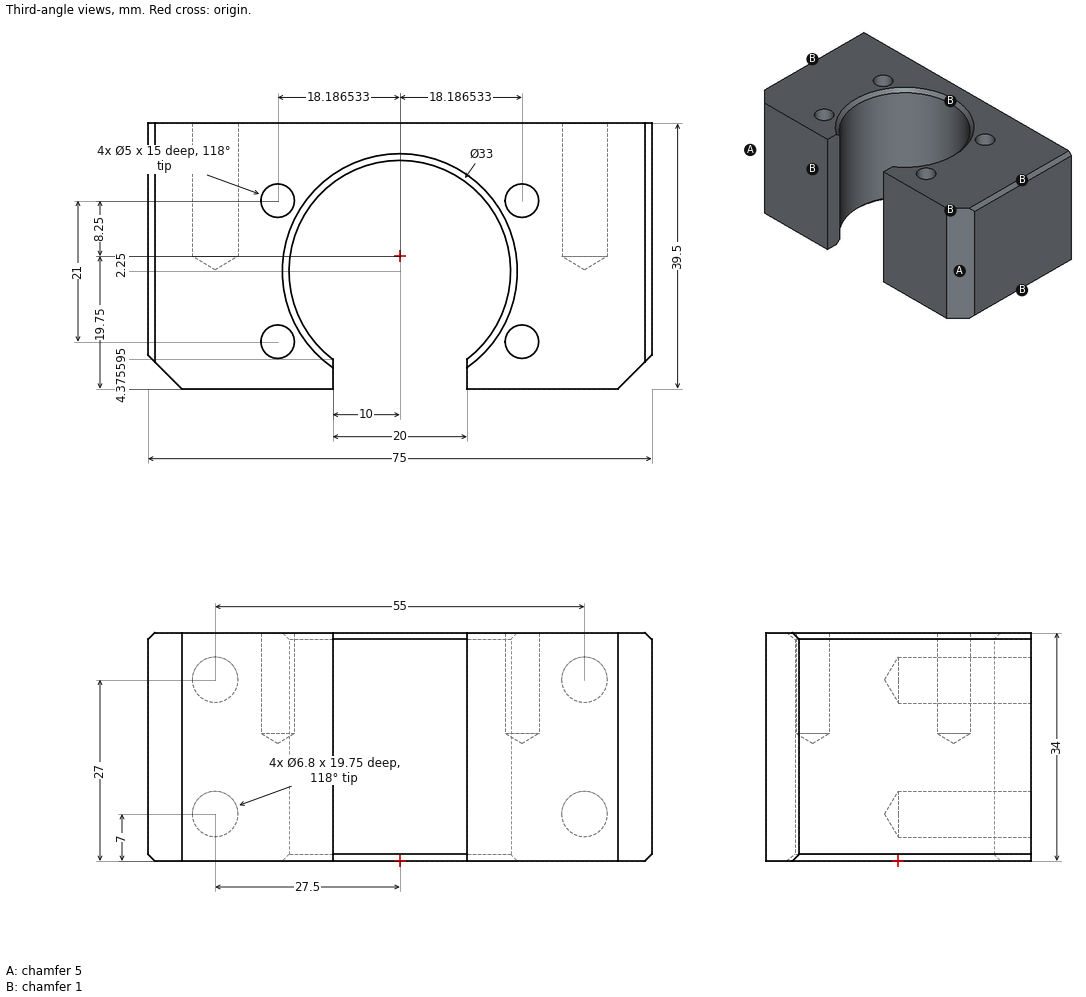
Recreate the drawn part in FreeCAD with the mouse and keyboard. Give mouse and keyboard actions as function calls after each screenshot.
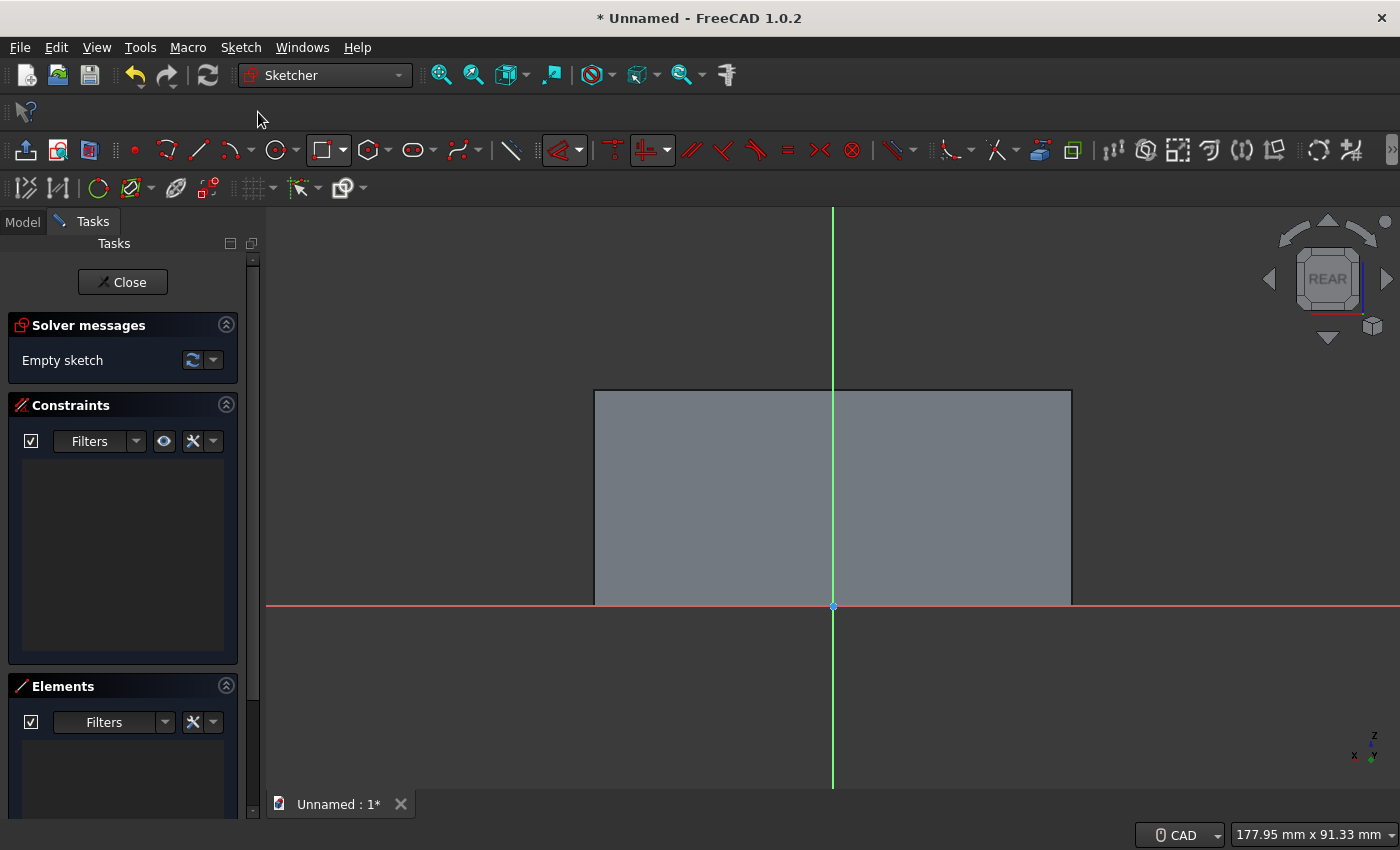
scroll(916, 523, up, 3)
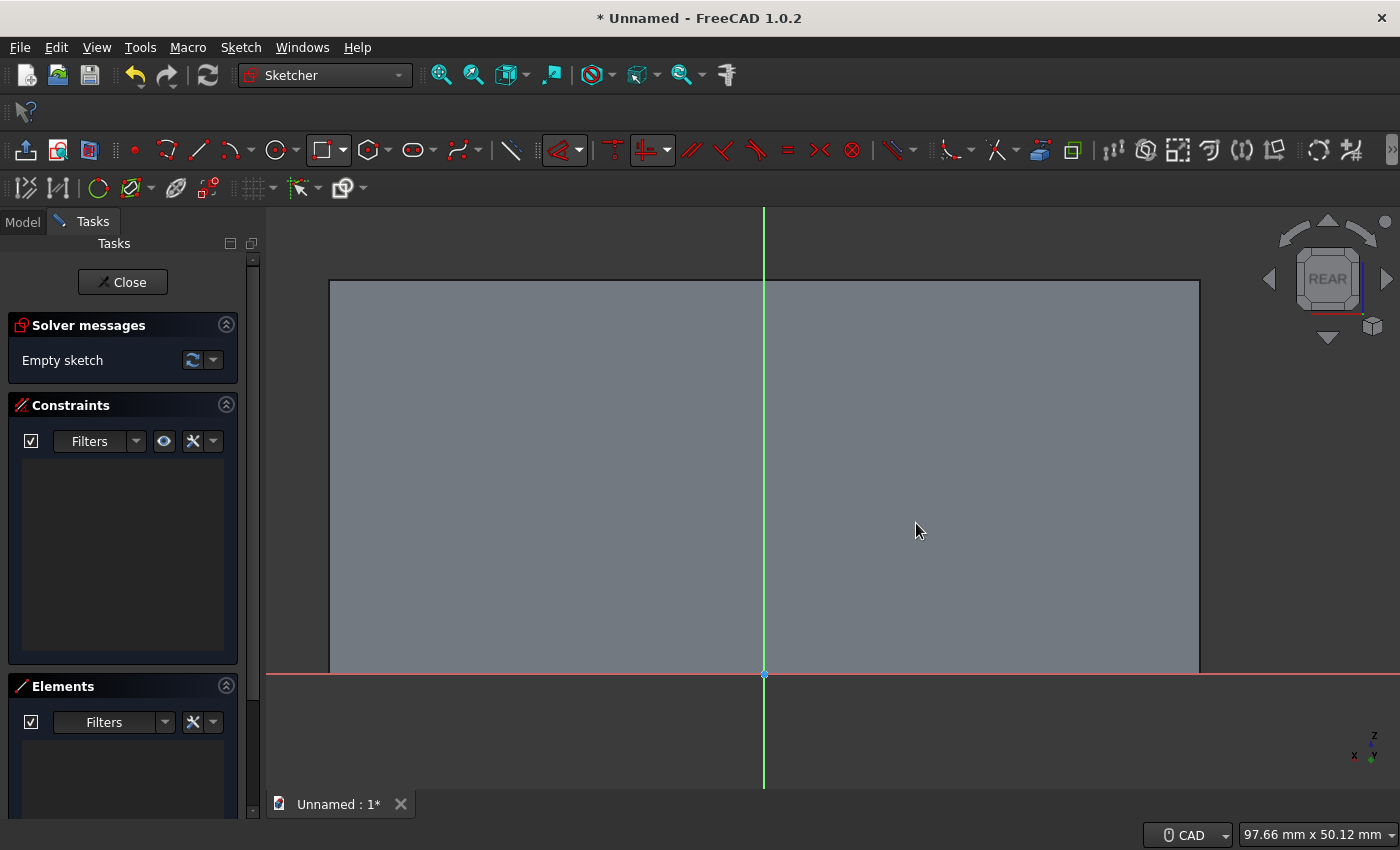
key(g)
key(c)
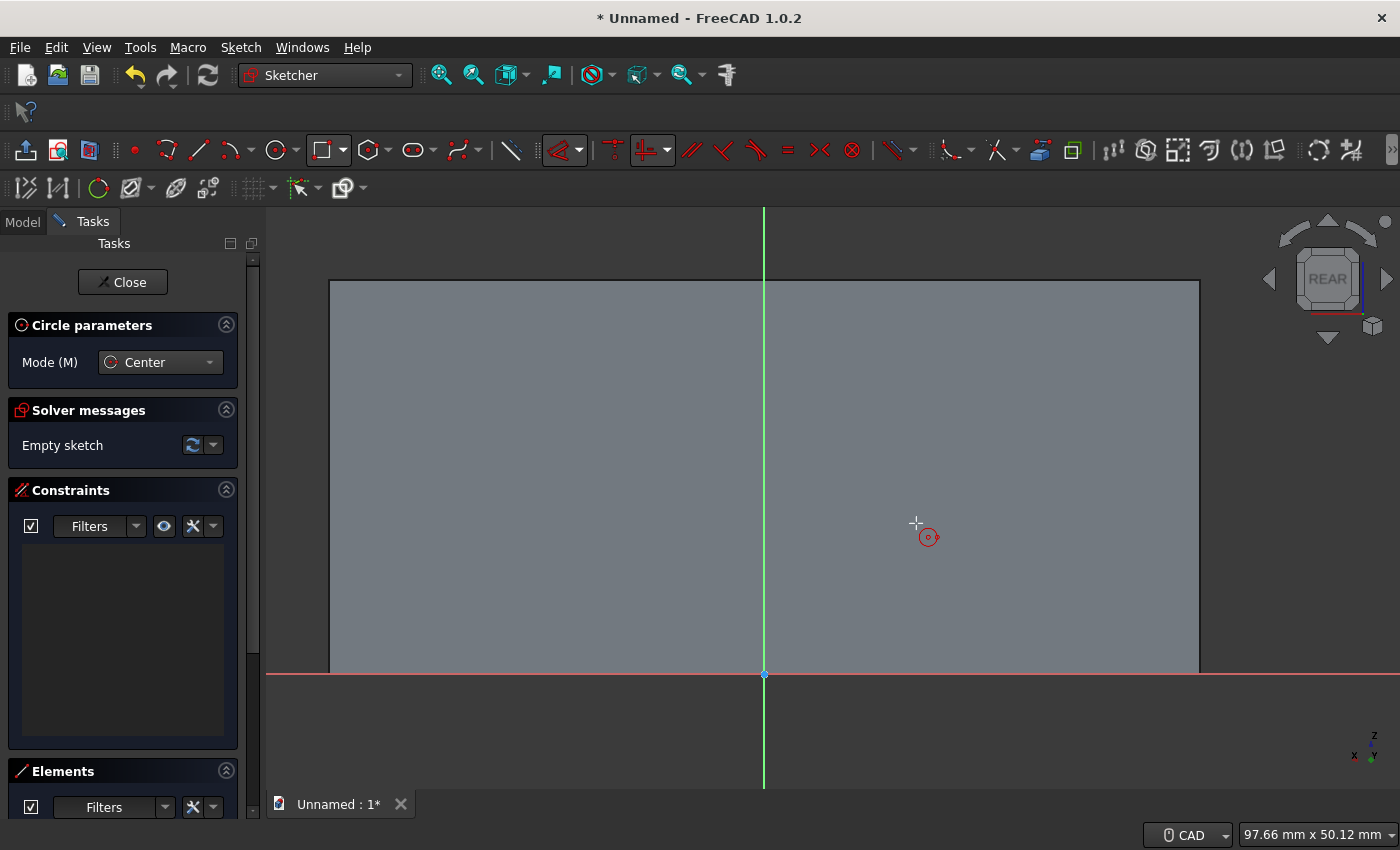
click(1084, 593)
click(1112, 565)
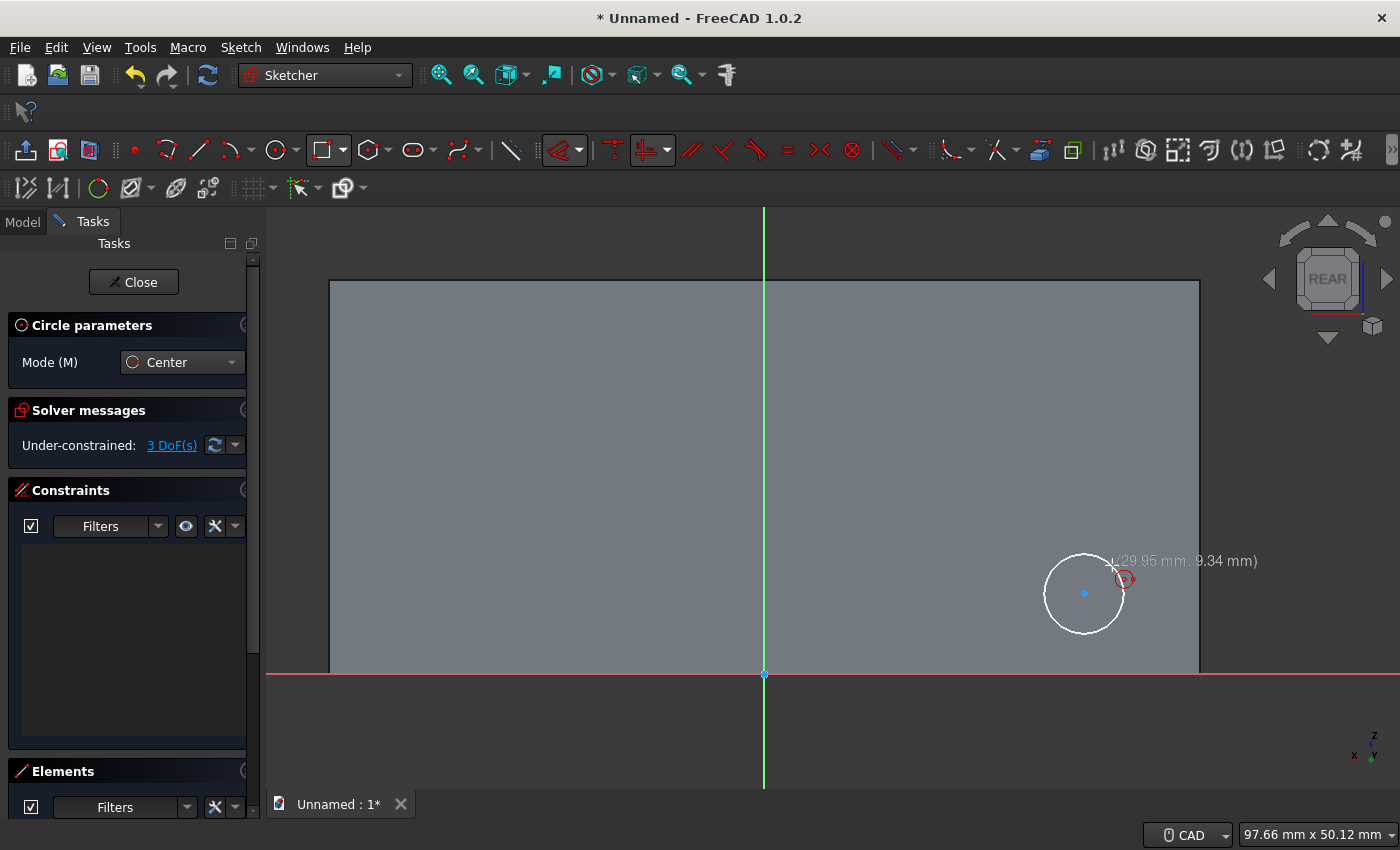
click(1084, 361)
click(1112, 333)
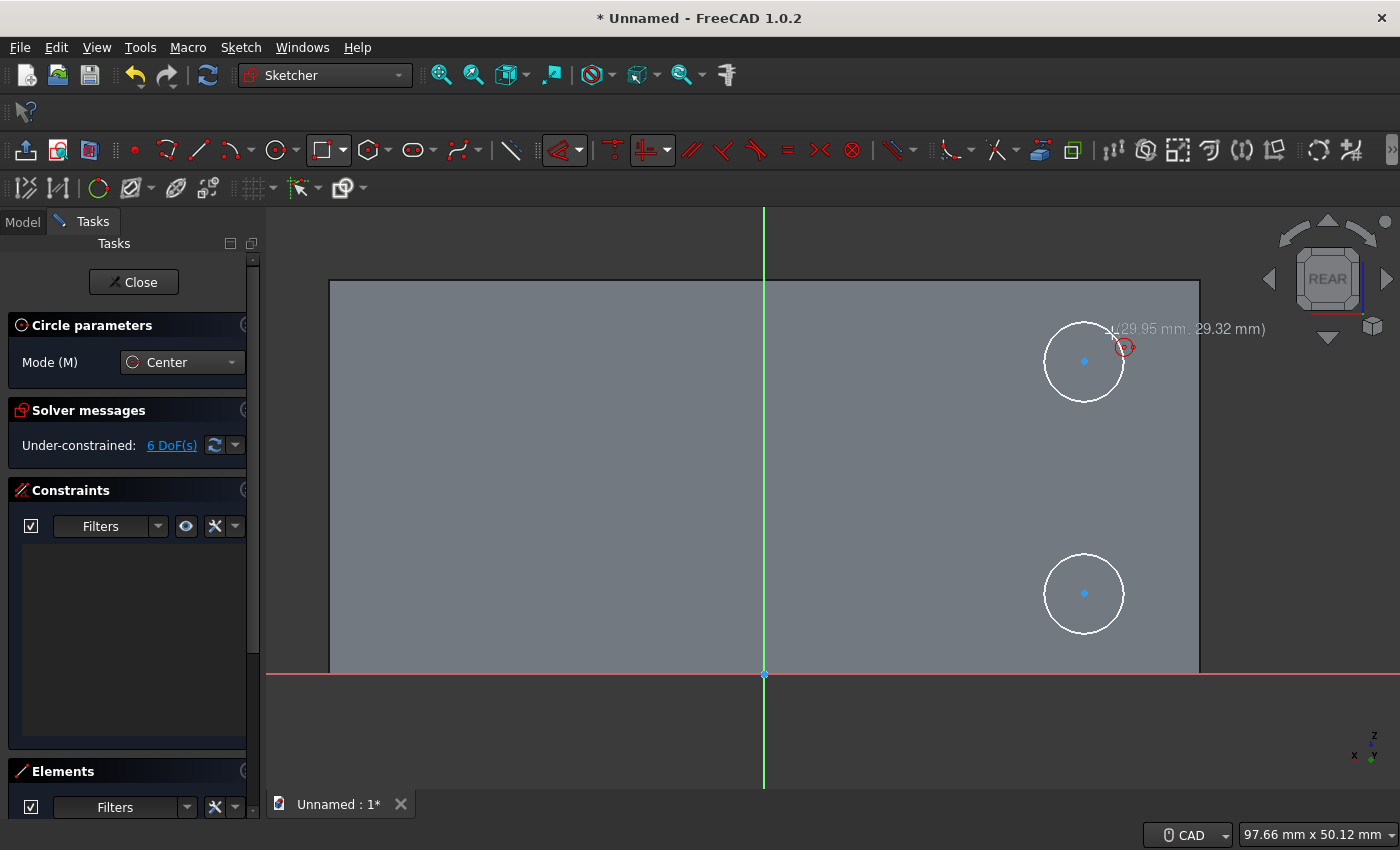
click(445, 361)
click(473, 333)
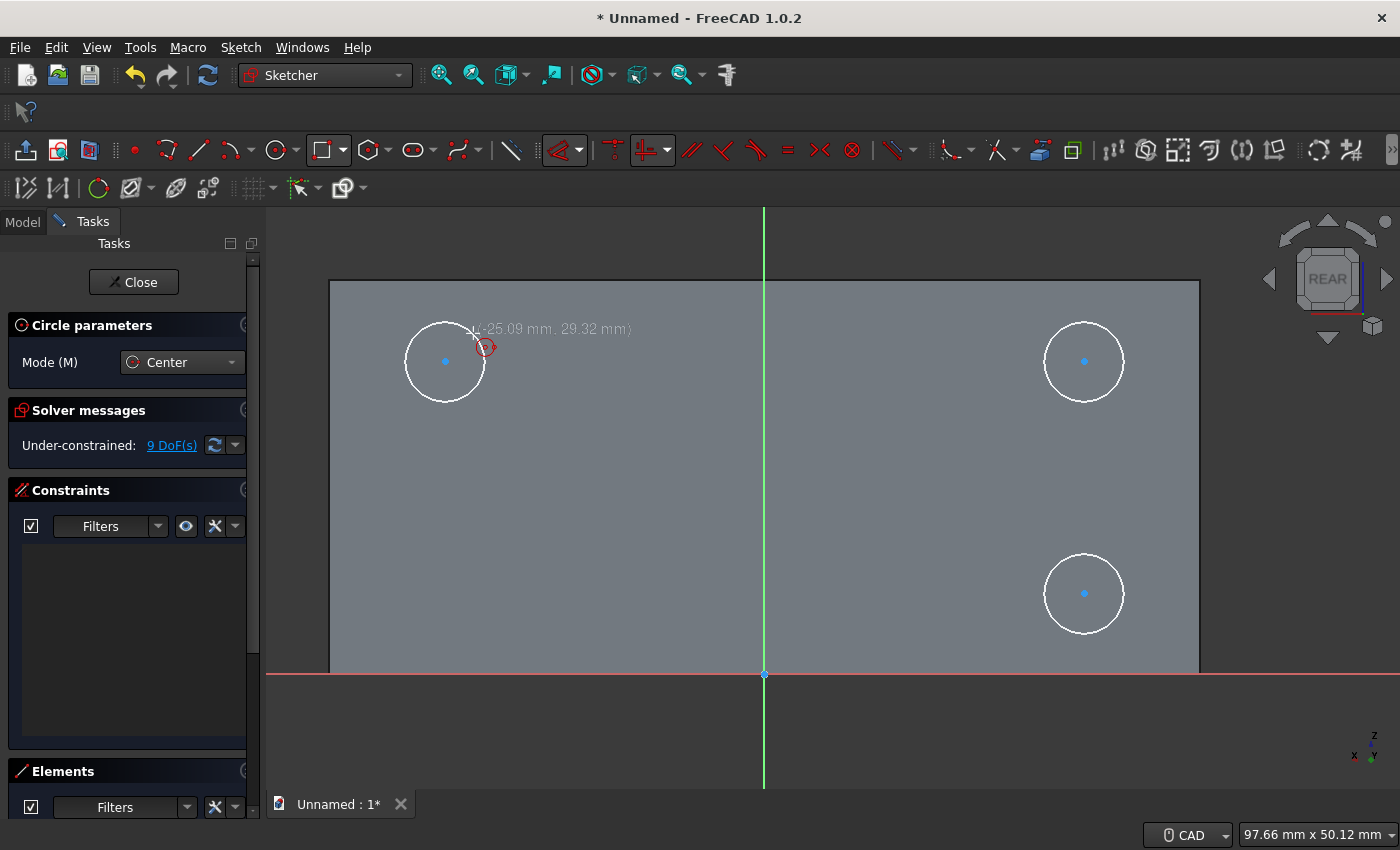
click(445, 593)
click(473, 565)
key(Escape)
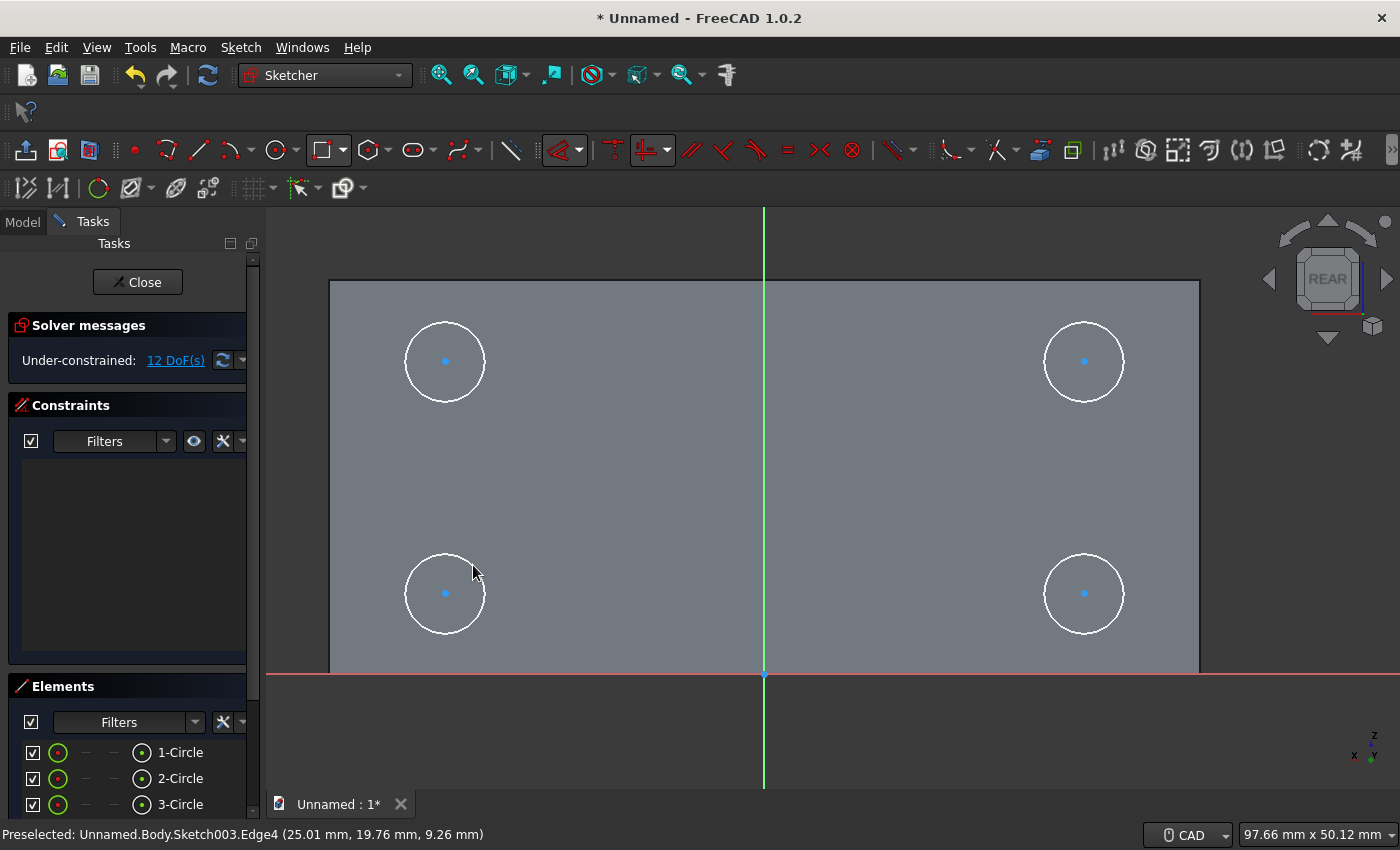
click(1112, 566)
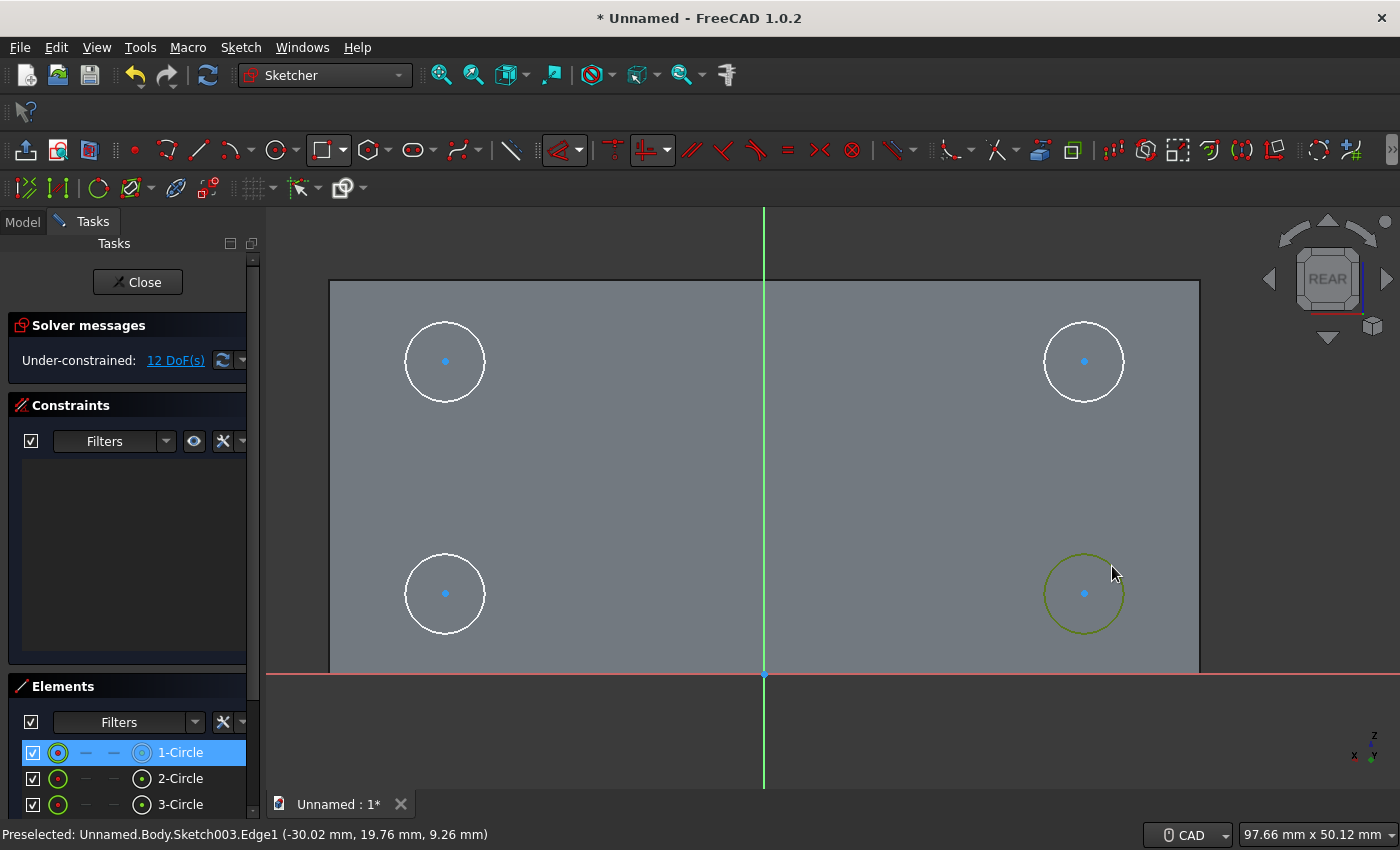
click(1112, 334)